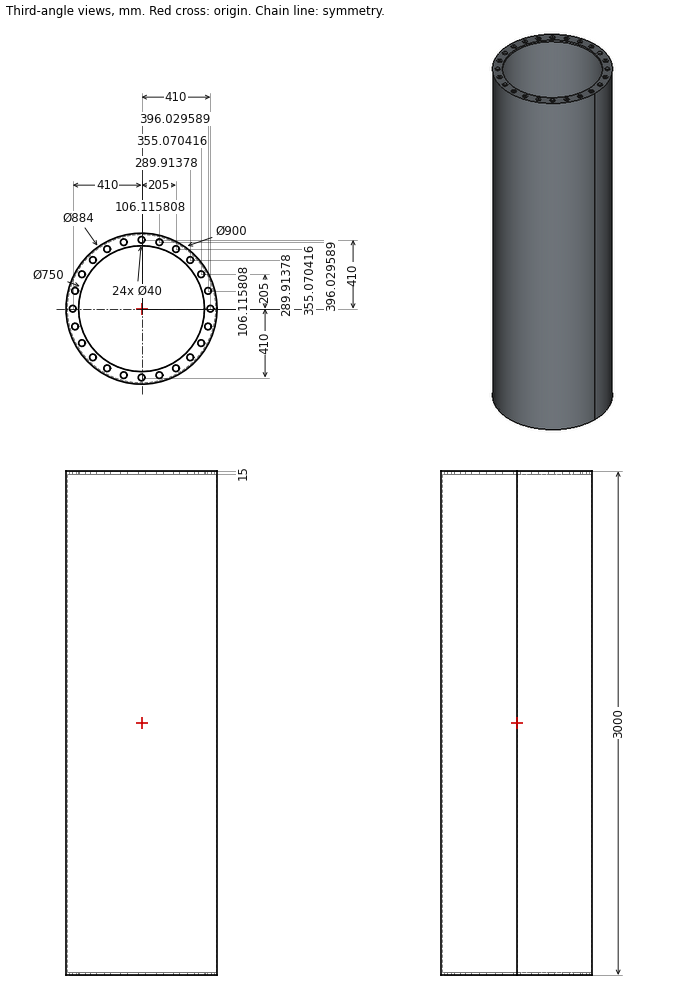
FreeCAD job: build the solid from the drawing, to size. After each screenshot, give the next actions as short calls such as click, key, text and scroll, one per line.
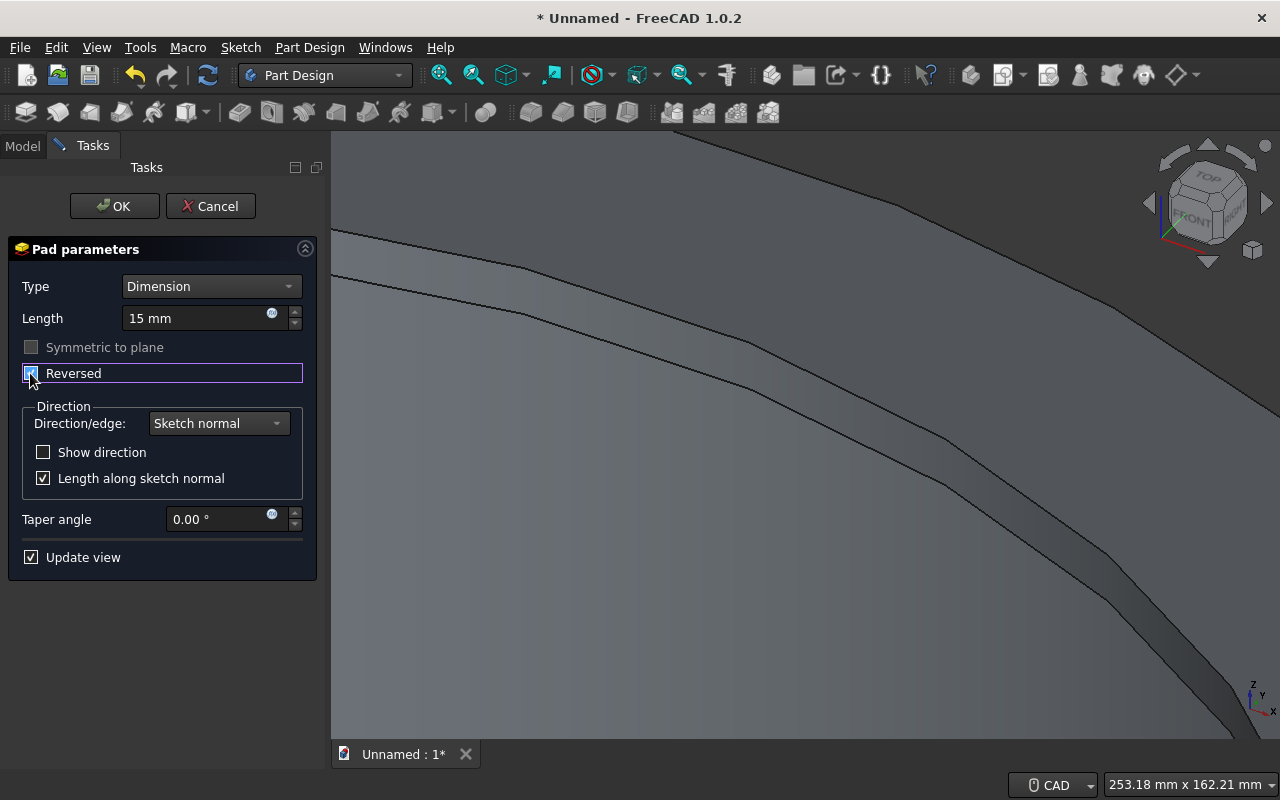
click(115, 206)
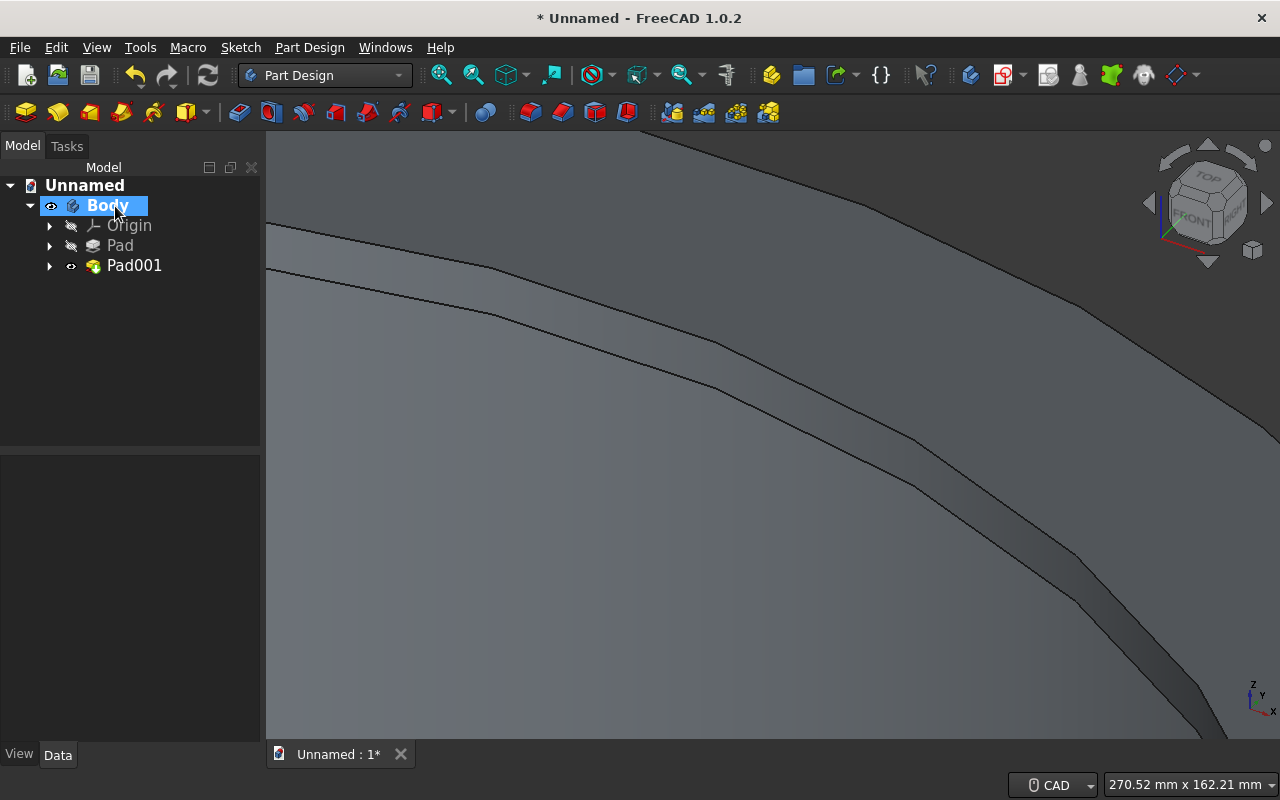
click(442, 76)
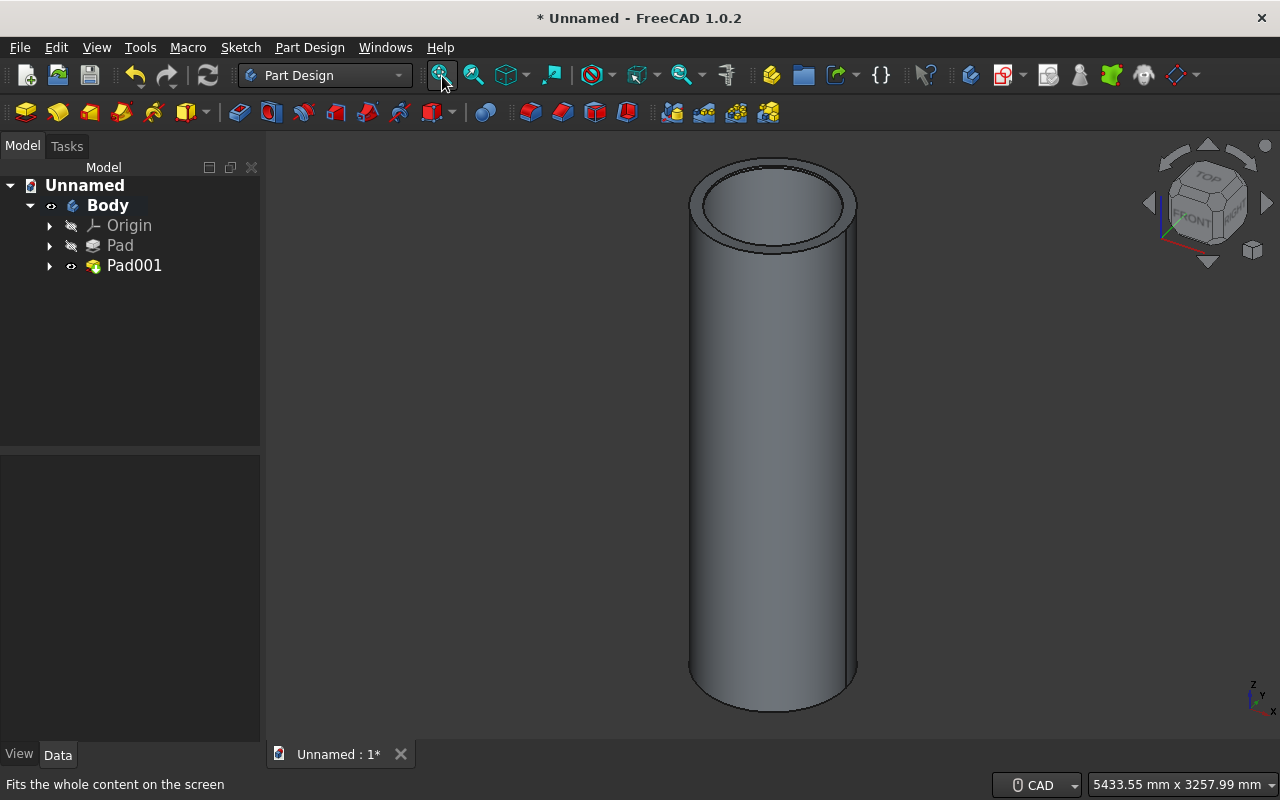
click(116, 266)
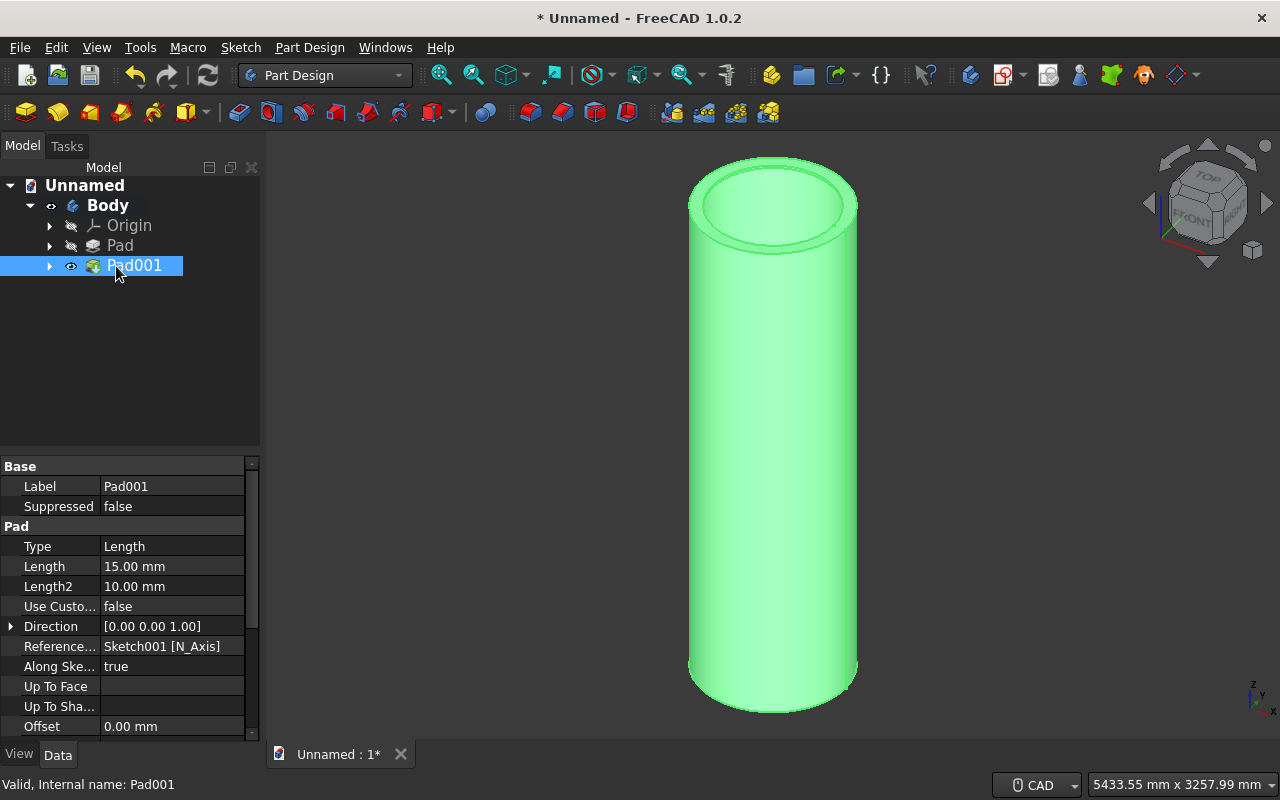
click(672, 112)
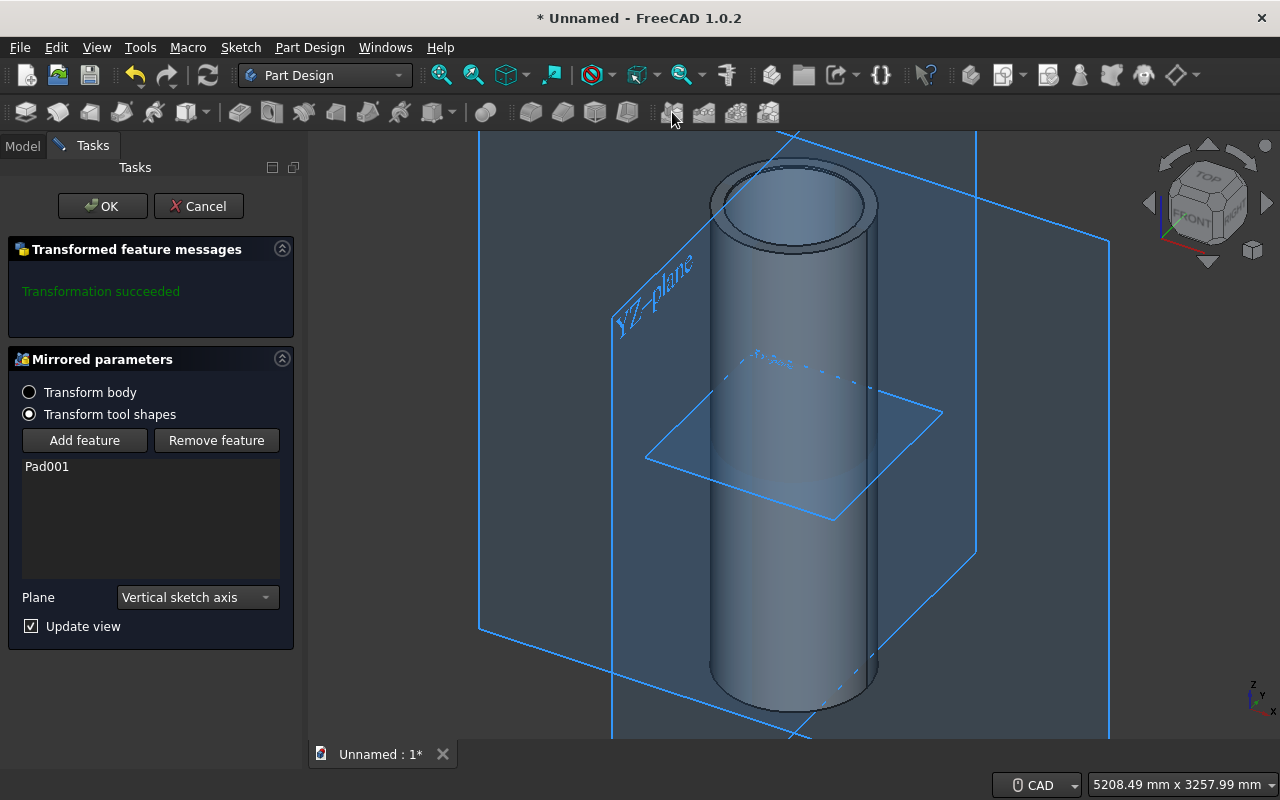
click(198, 598)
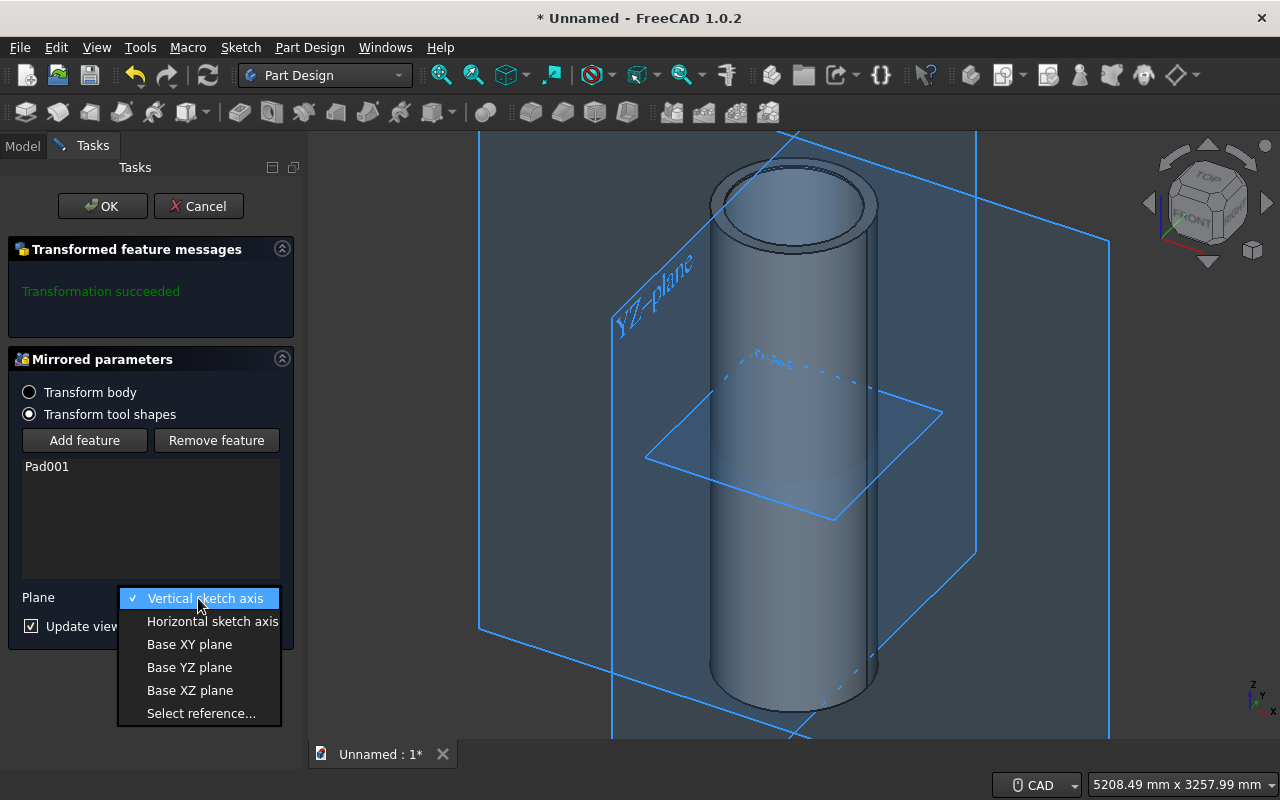
click(198, 644)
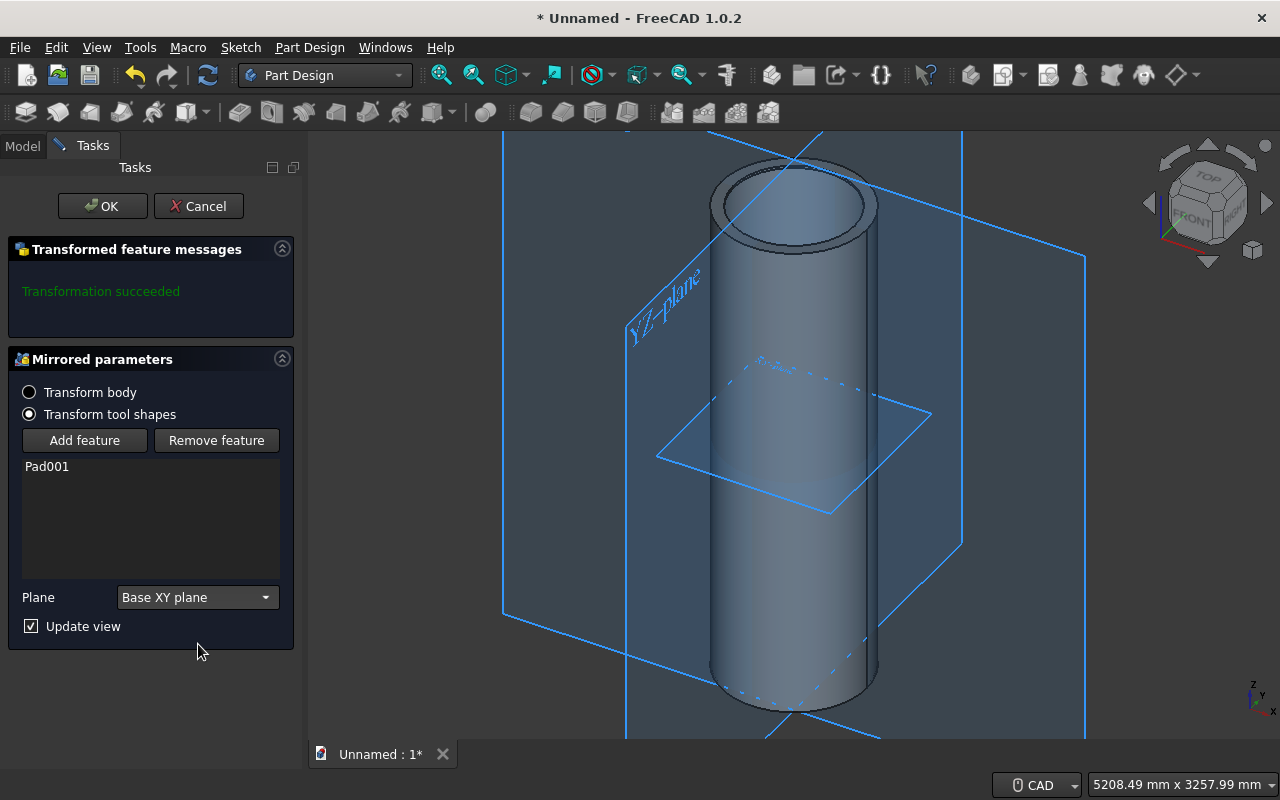
click(103, 206)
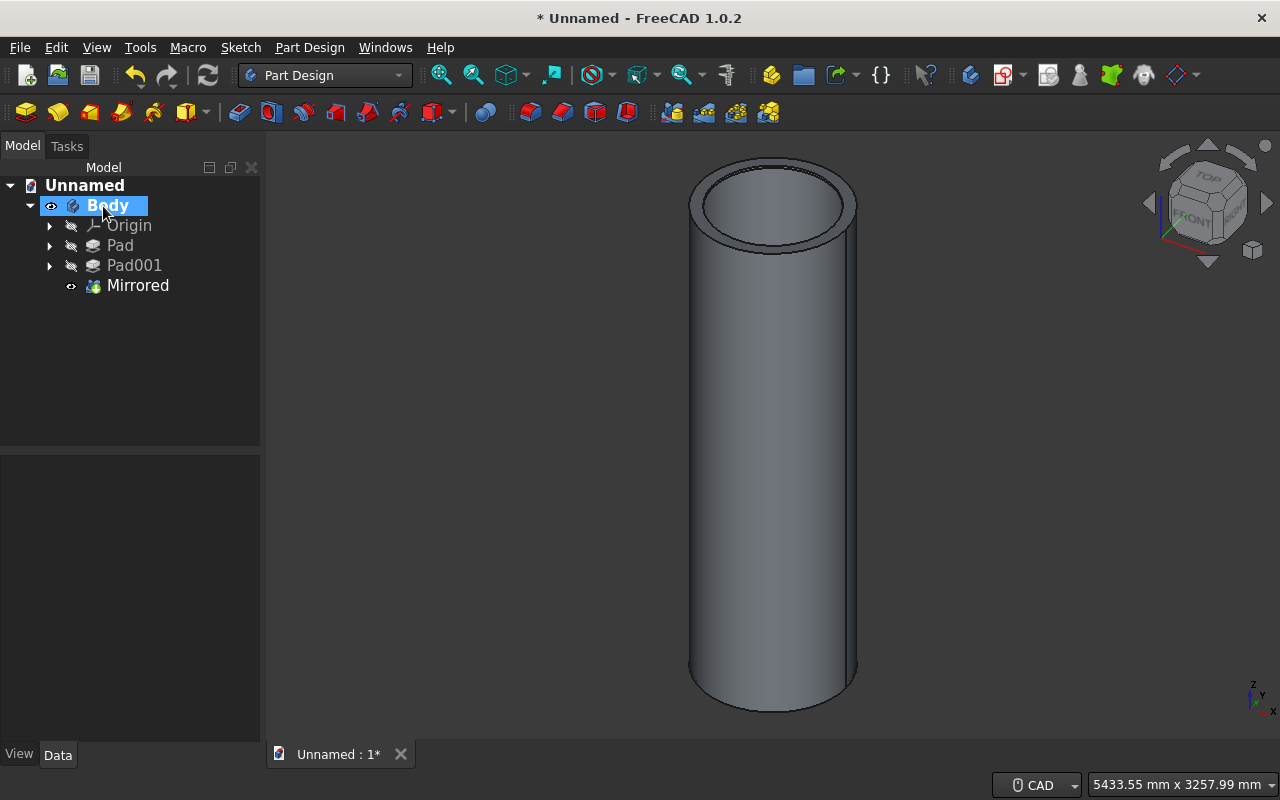
scroll(716, 234, up, 4)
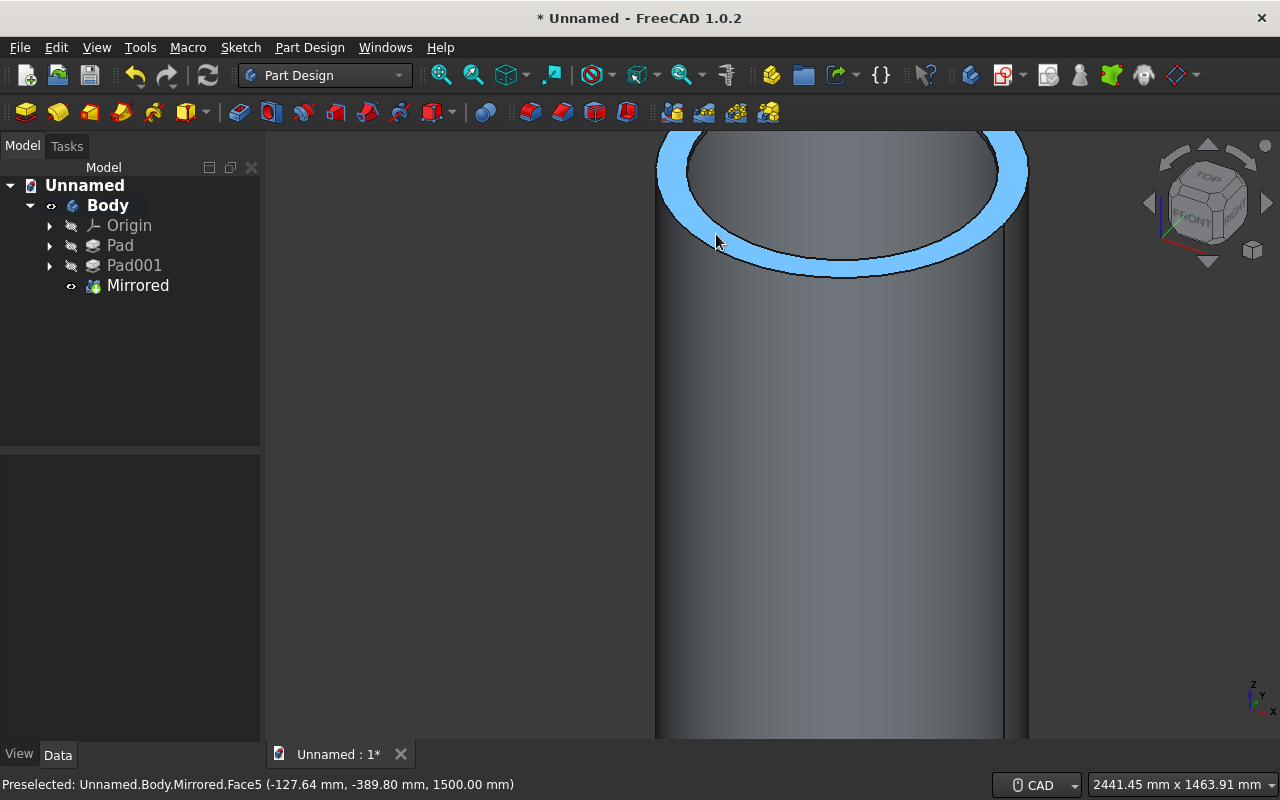
click(716, 234)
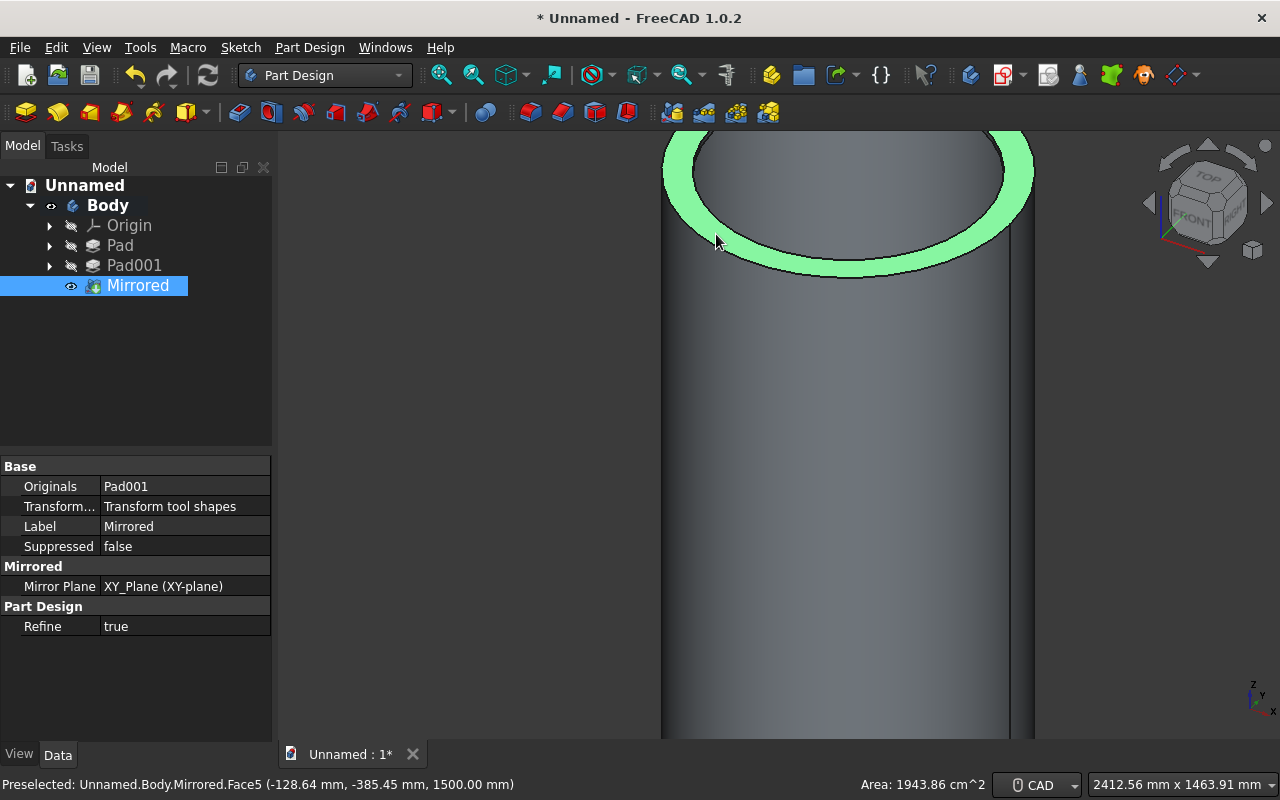
click(1004, 76)